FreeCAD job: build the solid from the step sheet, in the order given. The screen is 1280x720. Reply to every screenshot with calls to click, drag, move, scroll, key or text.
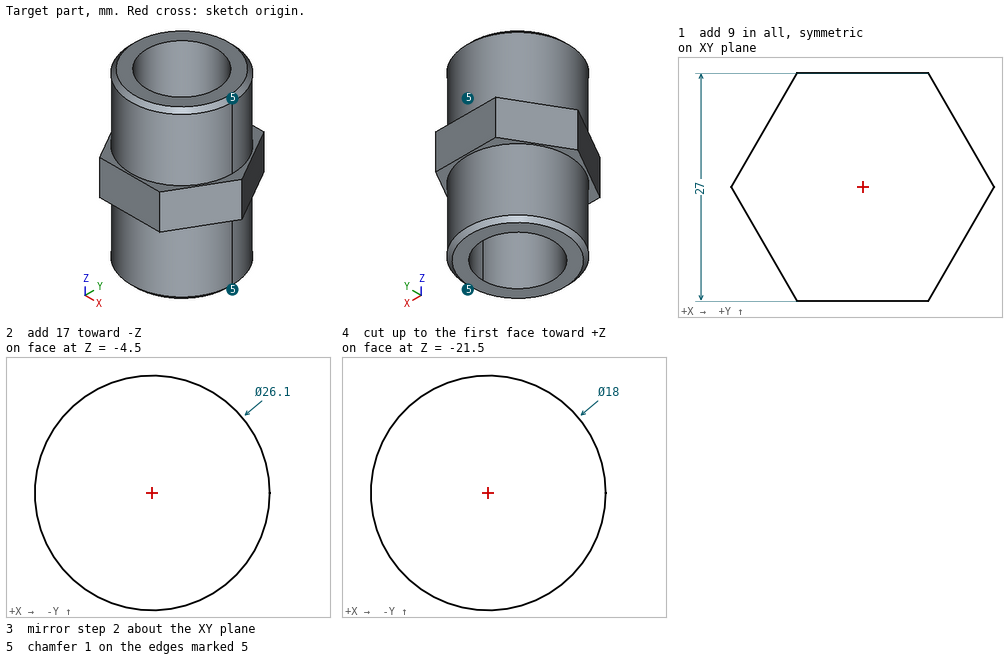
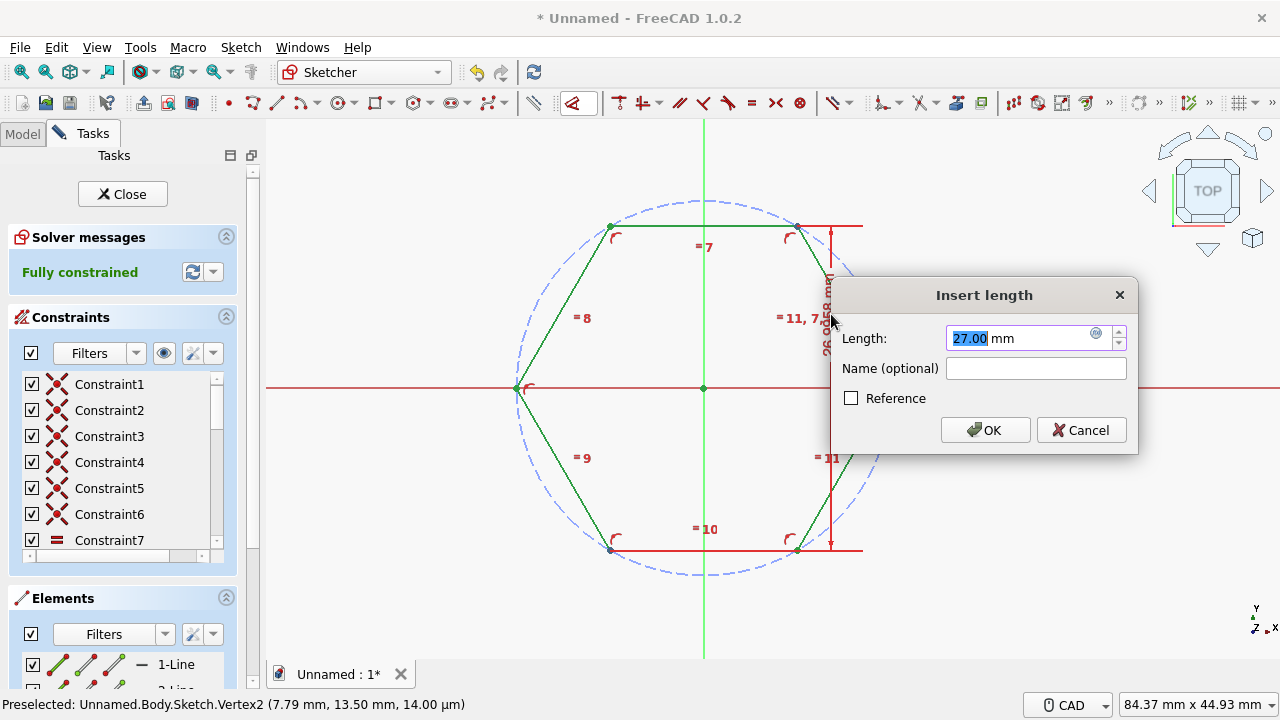
text(27)
key(Return)
key(Escape)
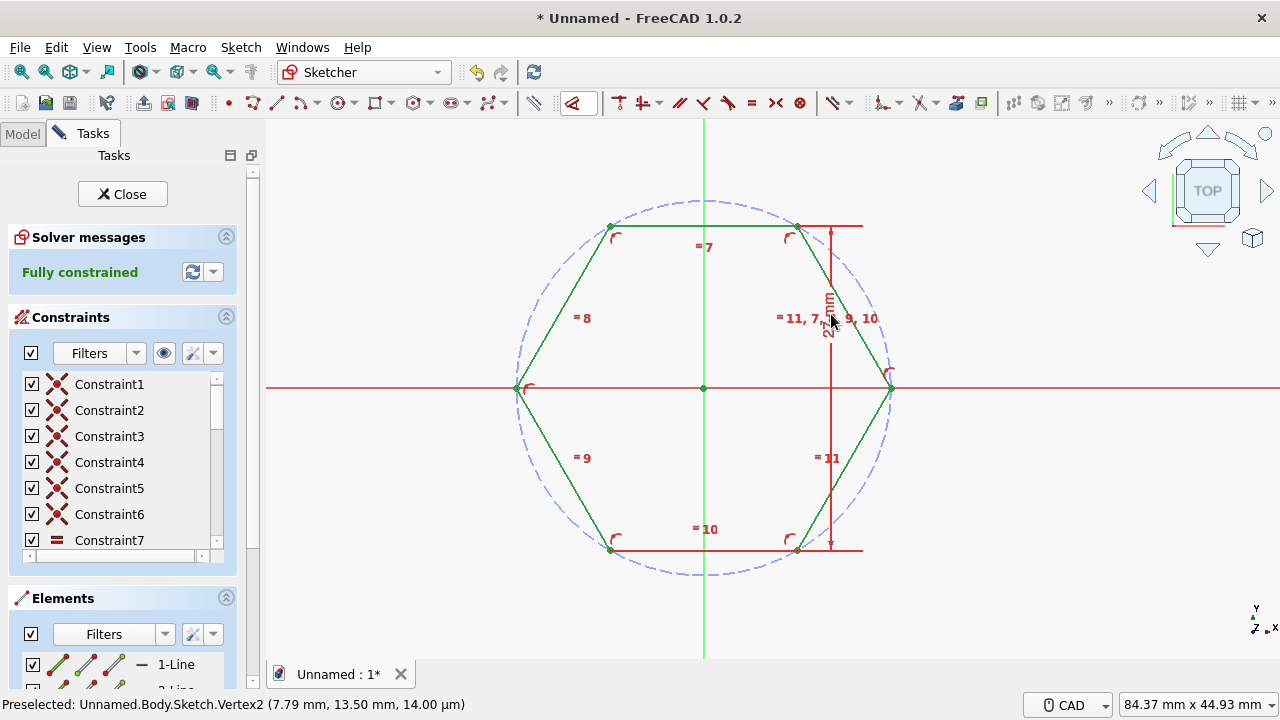
click(123, 194)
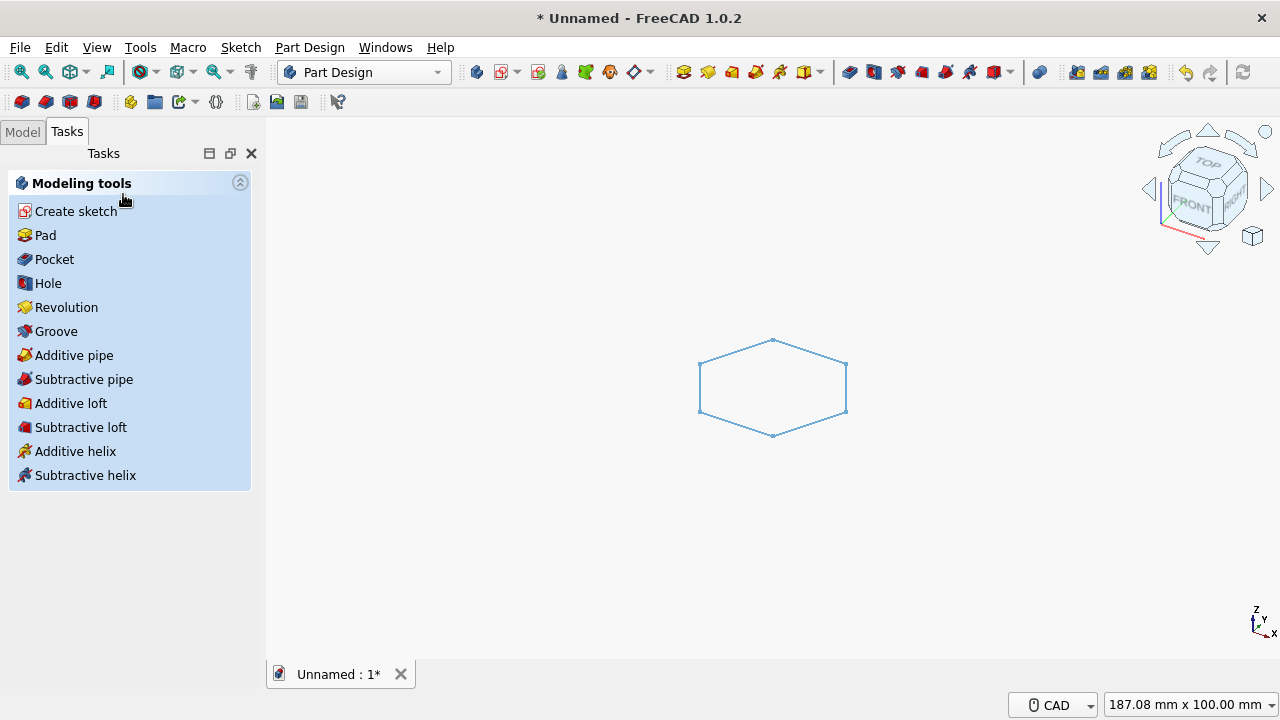
click(684, 72)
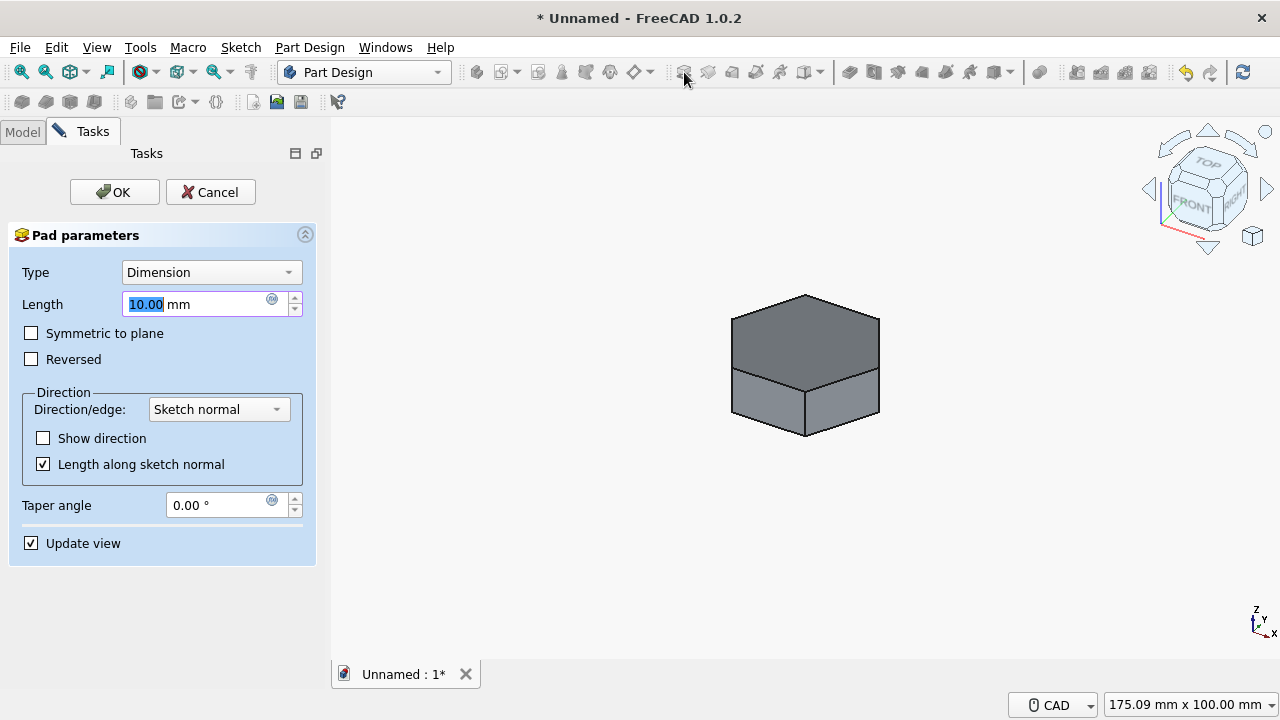
text(9)
key(Tab)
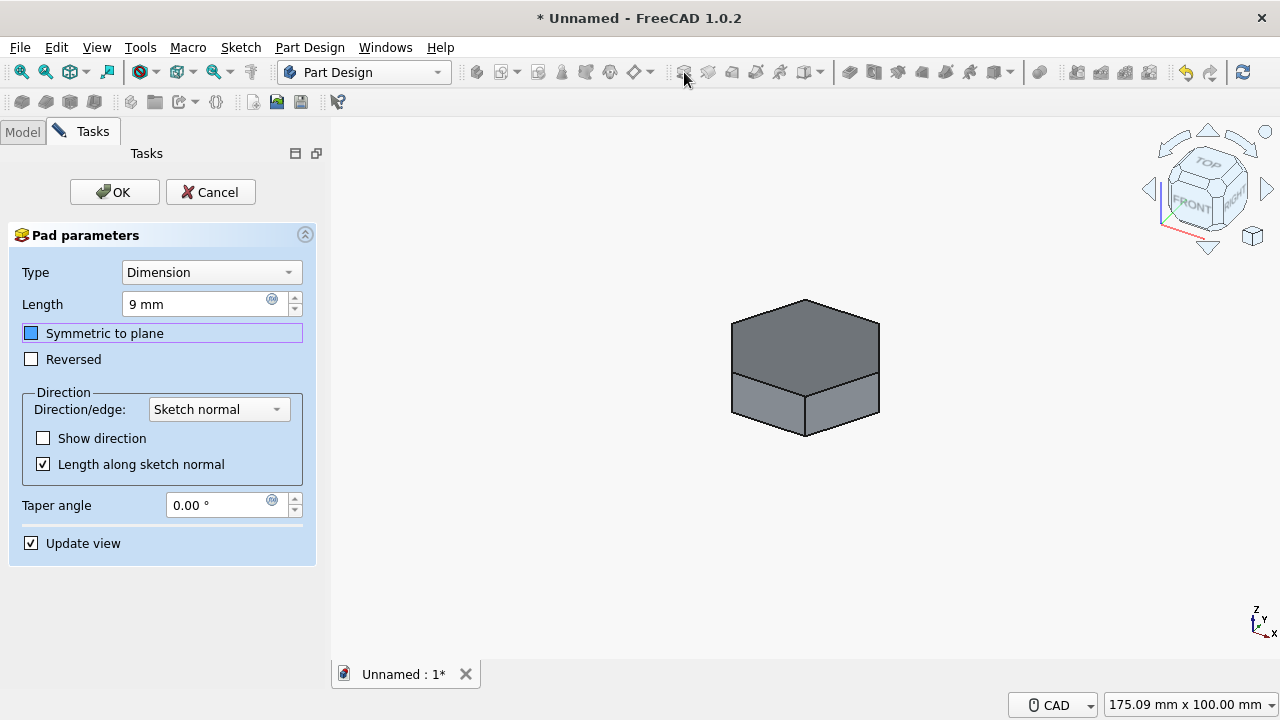
click(30, 333)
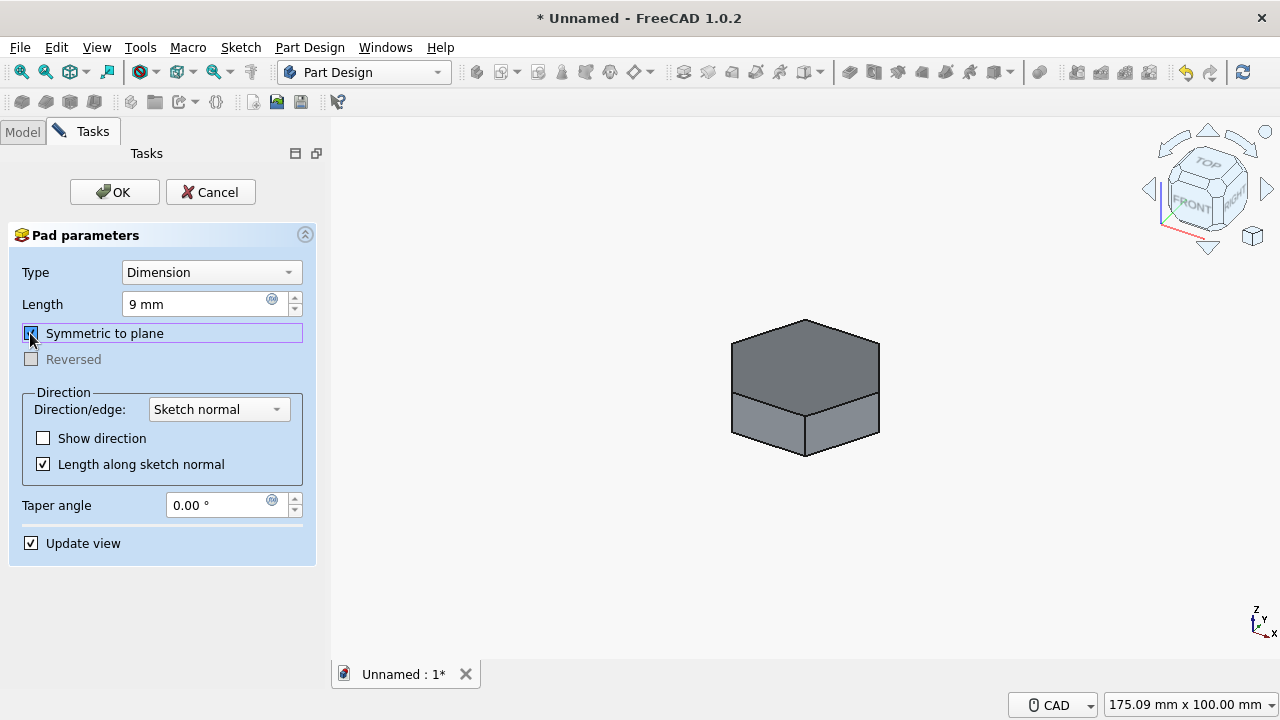
click(115, 192)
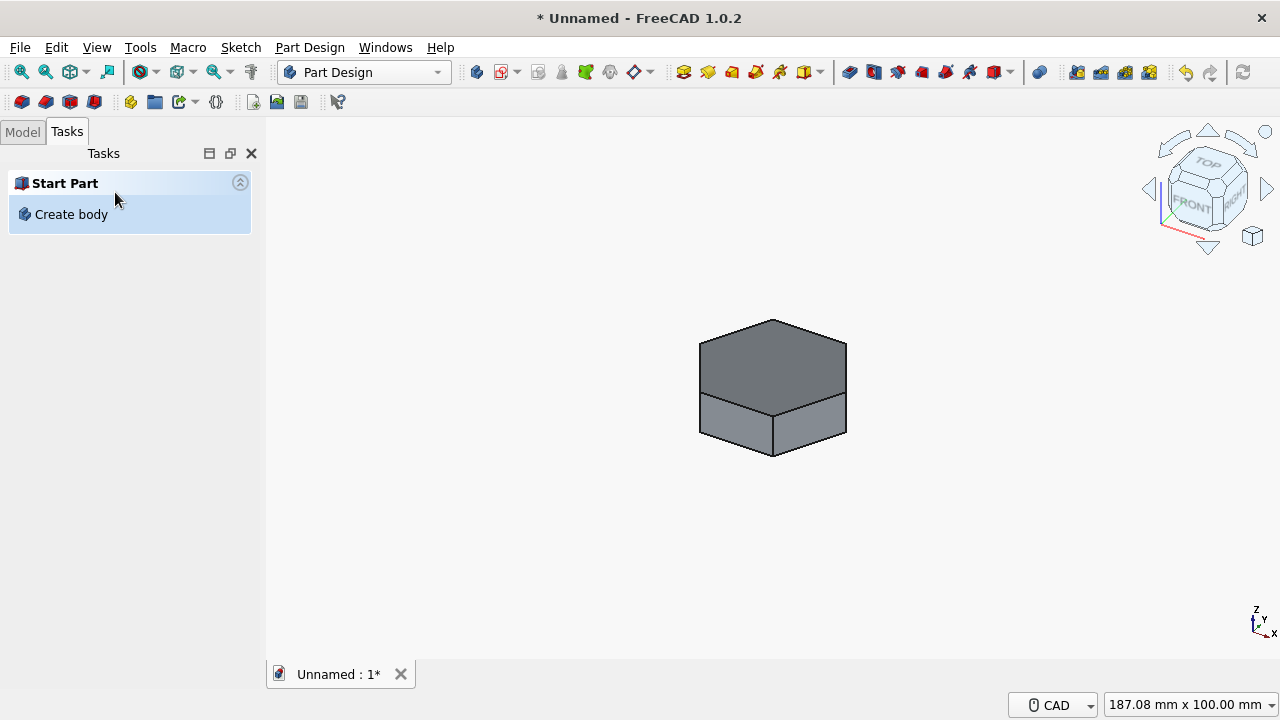
key(v)
key(f)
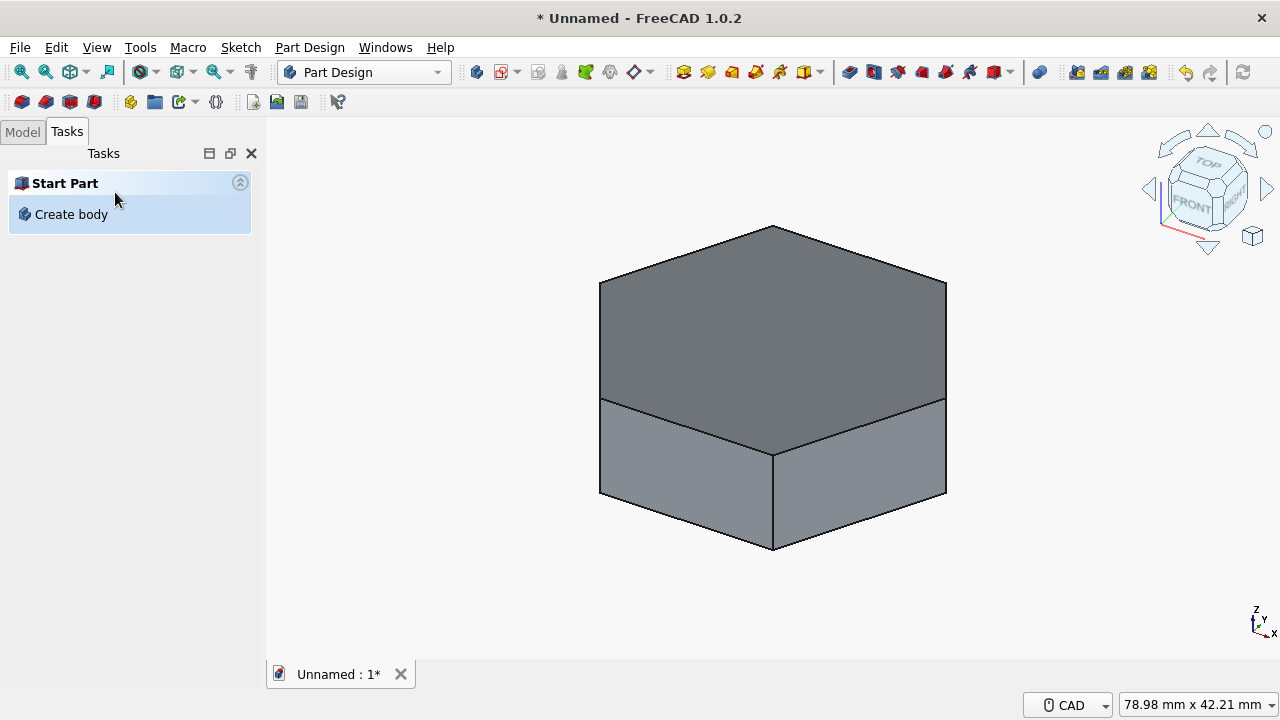
key(5)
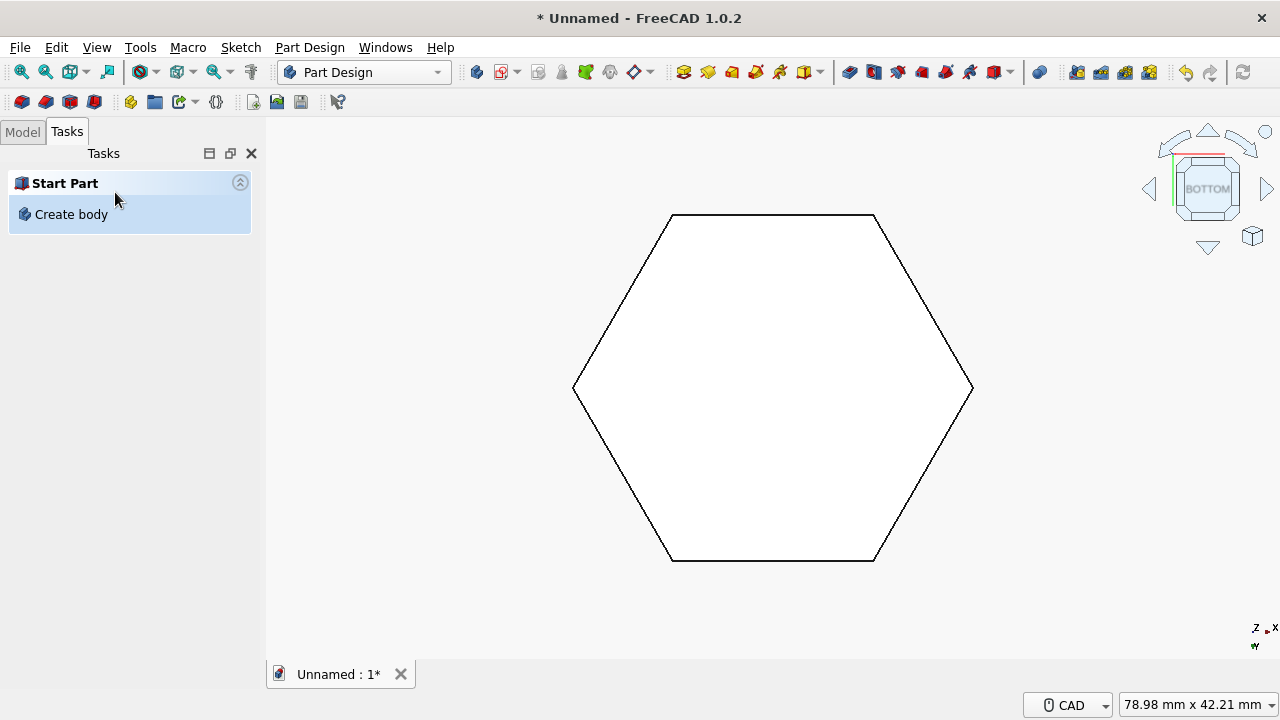
click(773, 387)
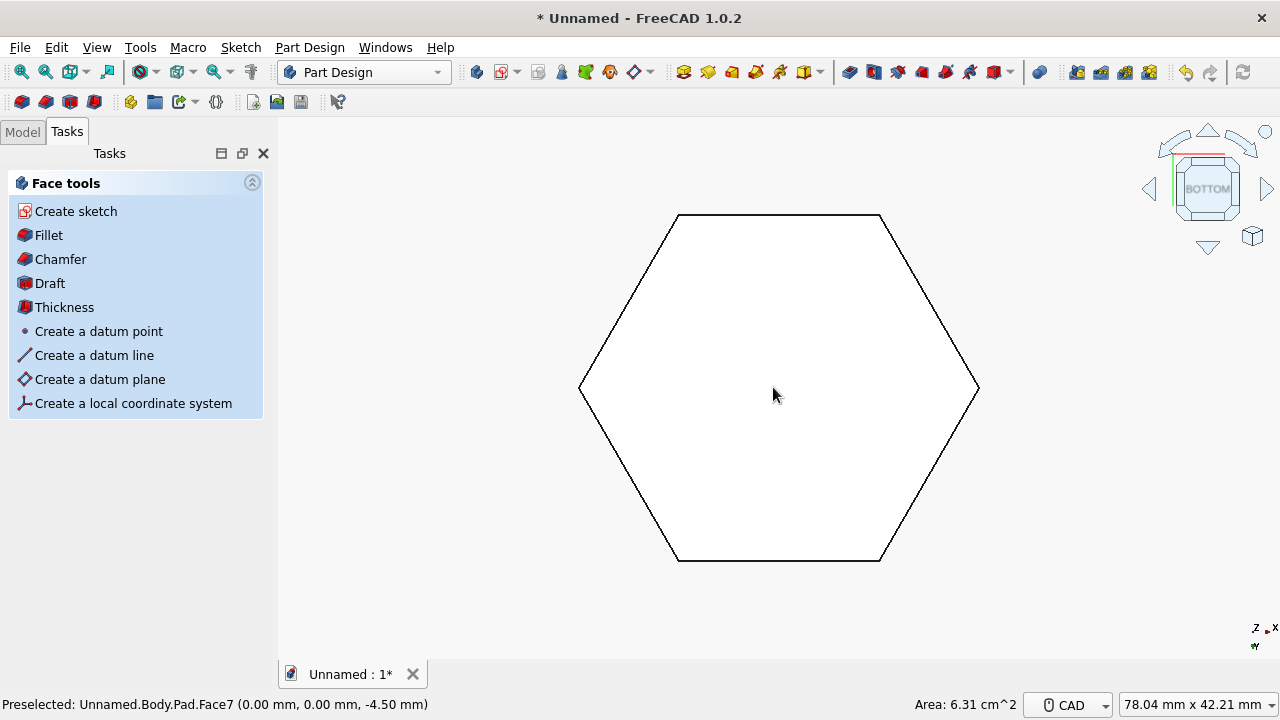
click(502, 72)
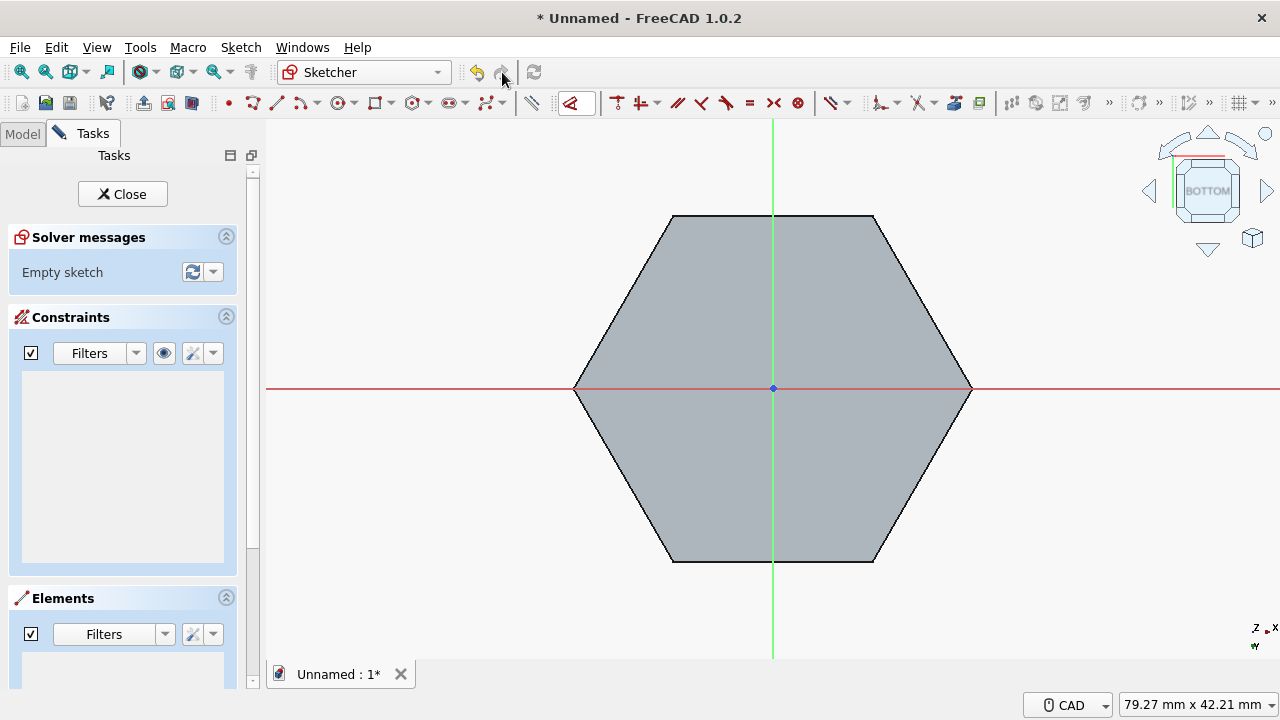
key(g)
key(c)